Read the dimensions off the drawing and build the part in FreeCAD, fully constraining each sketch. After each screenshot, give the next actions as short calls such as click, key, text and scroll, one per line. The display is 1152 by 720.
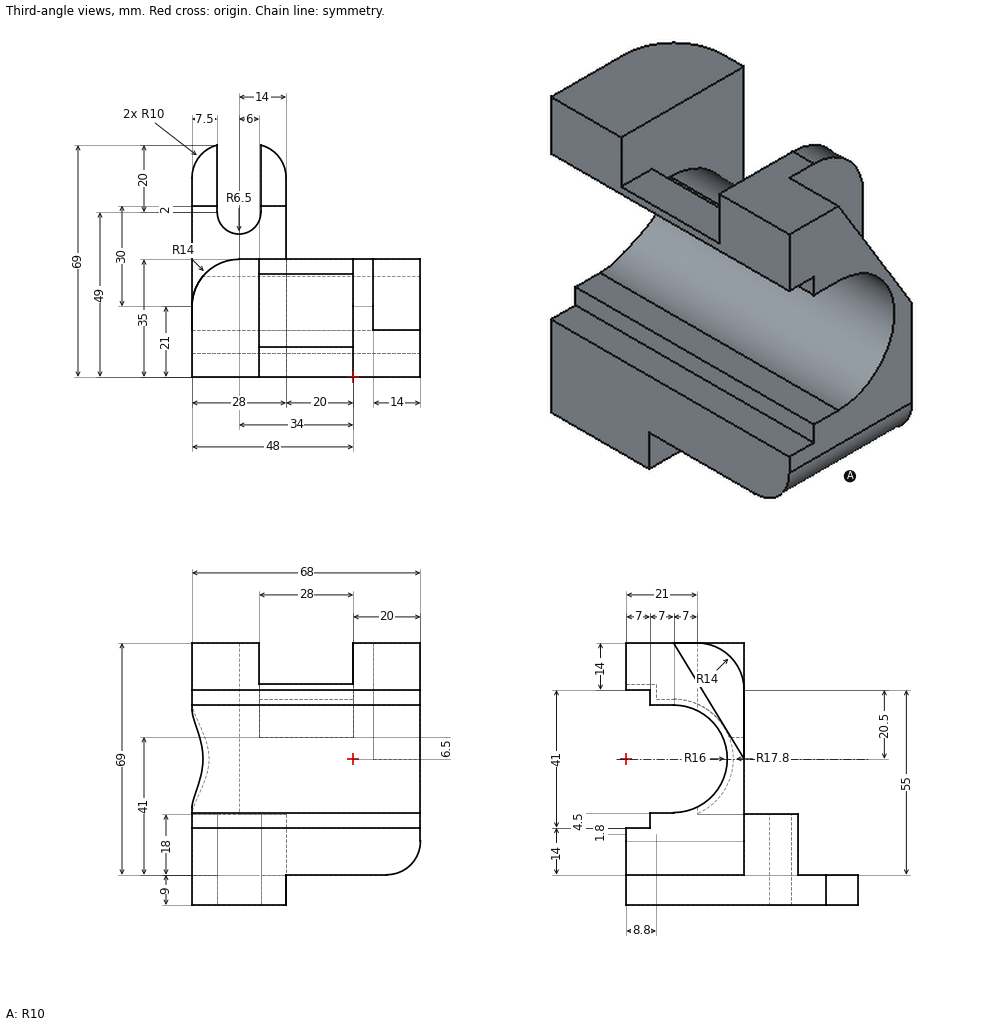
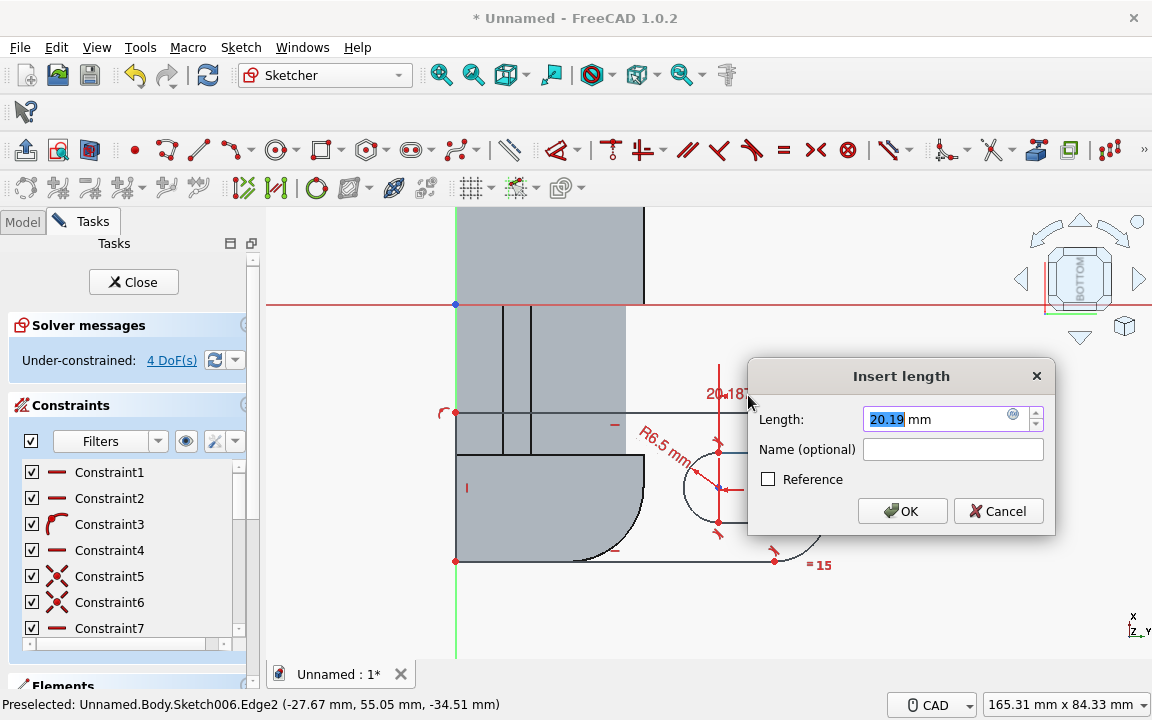
text(20)
key(Return)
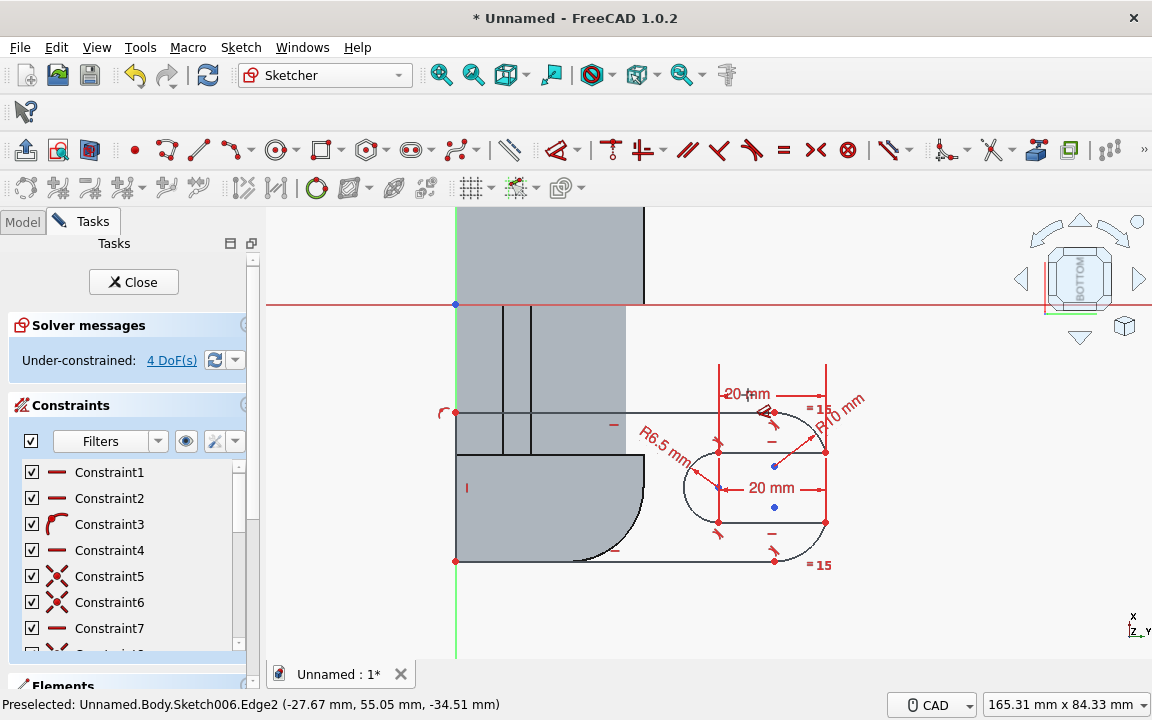
click(456, 458)
click(422, 487)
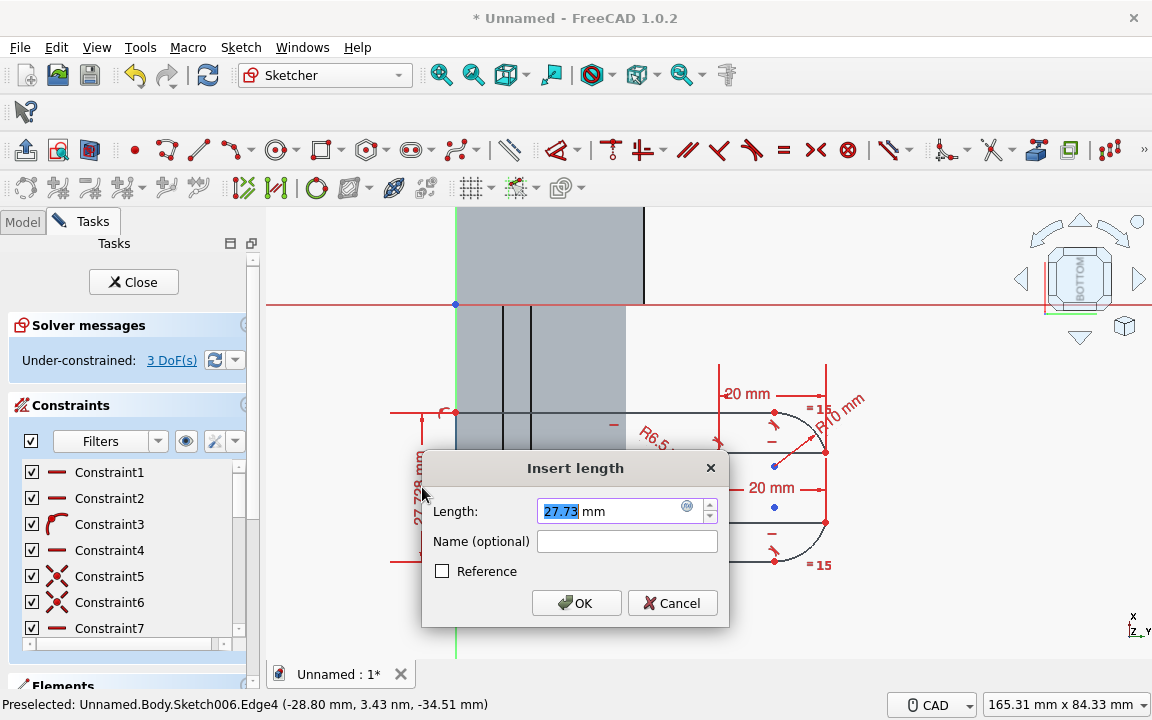
text(28)
key(Return)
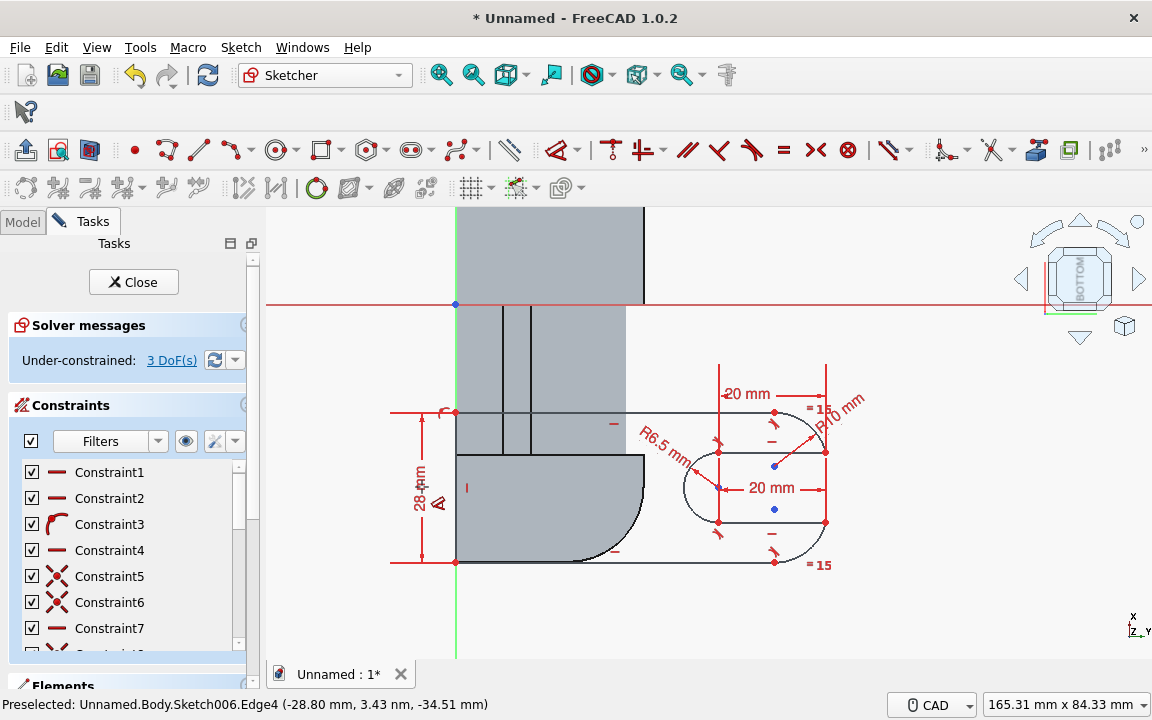
click(826, 523)
click(641, 271)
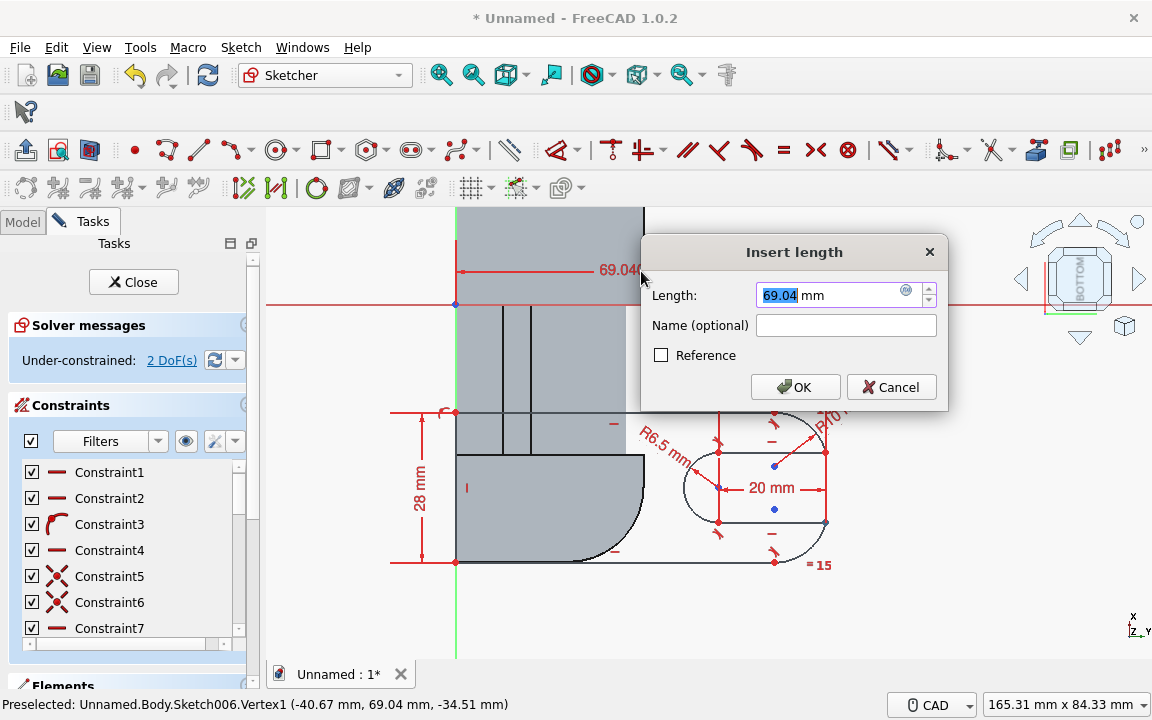
text(69)
key(Return)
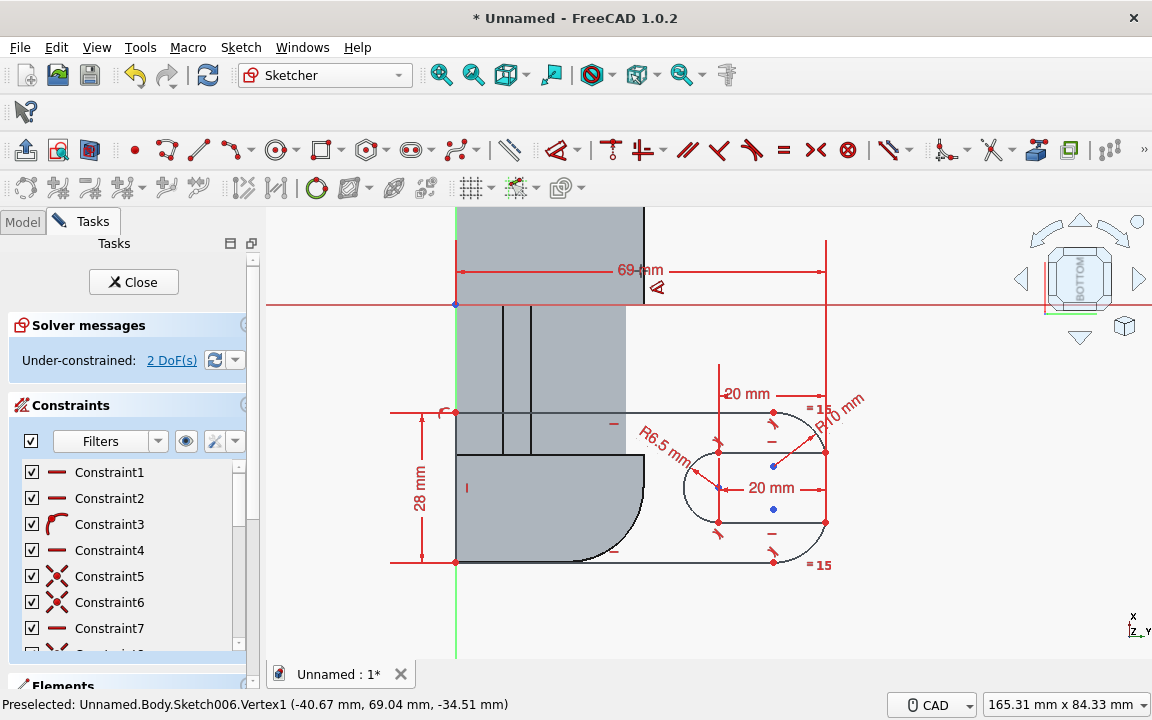
click(774, 413)
click(422, 359)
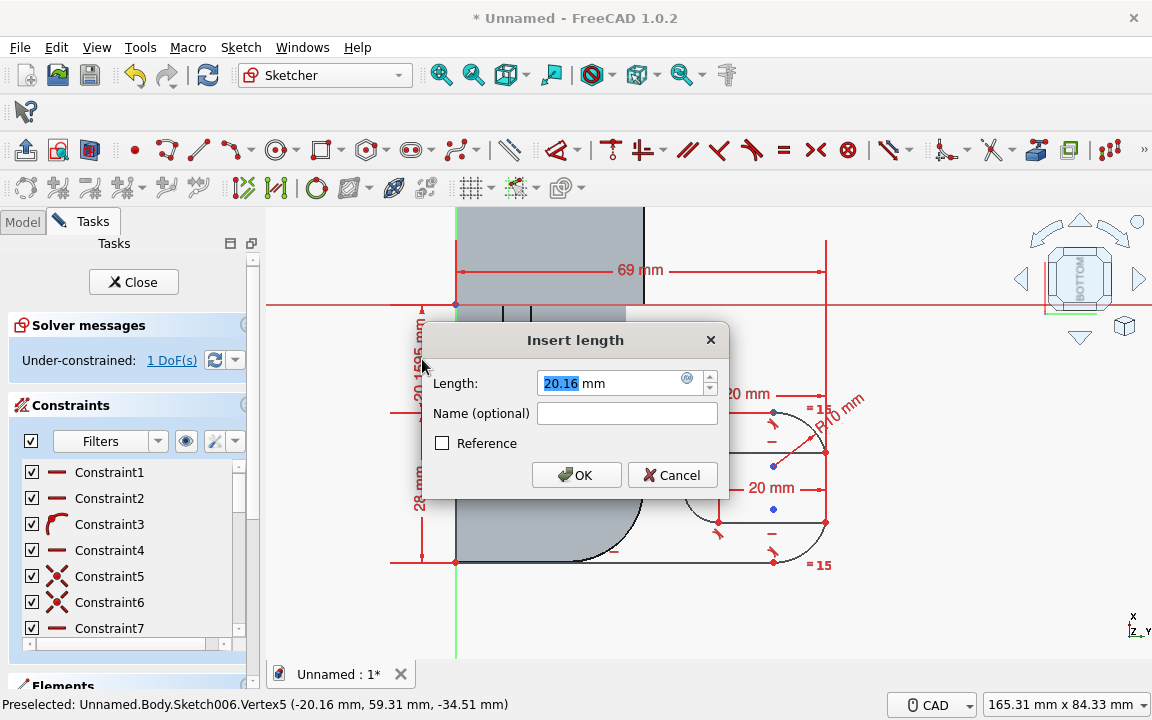
text(20)
key(Return)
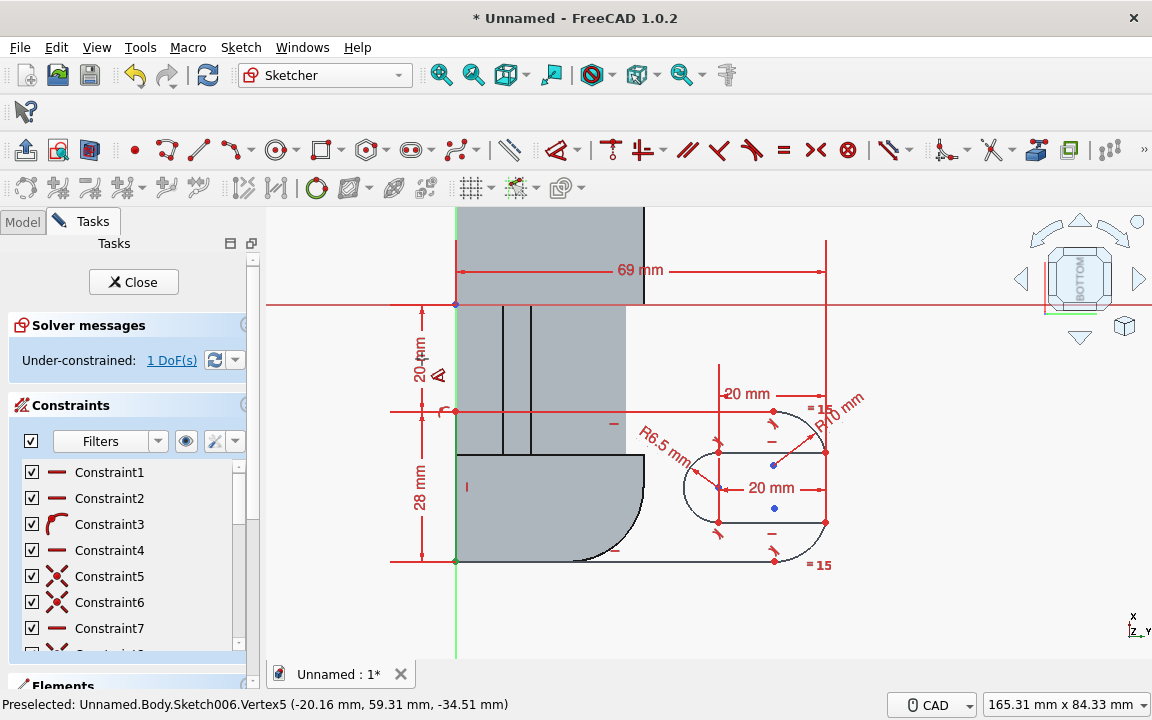
click(719, 488)
click(422, 396)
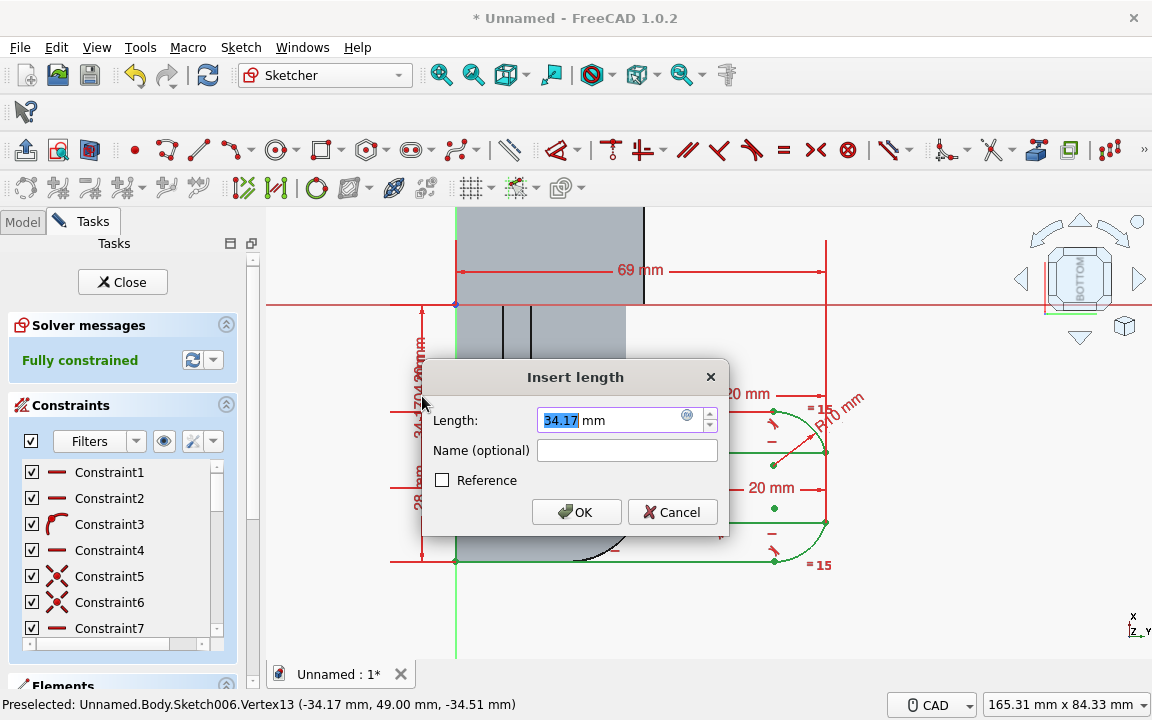
text(34)
key(Return)
key(Escape)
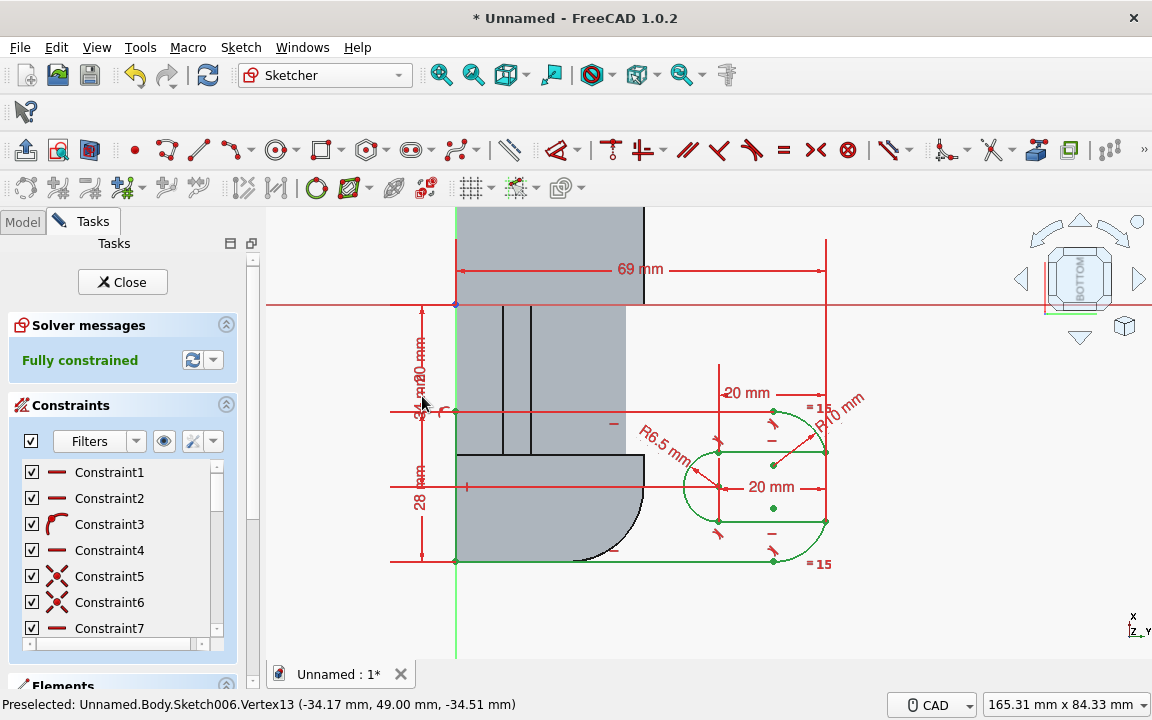
click(123, 282)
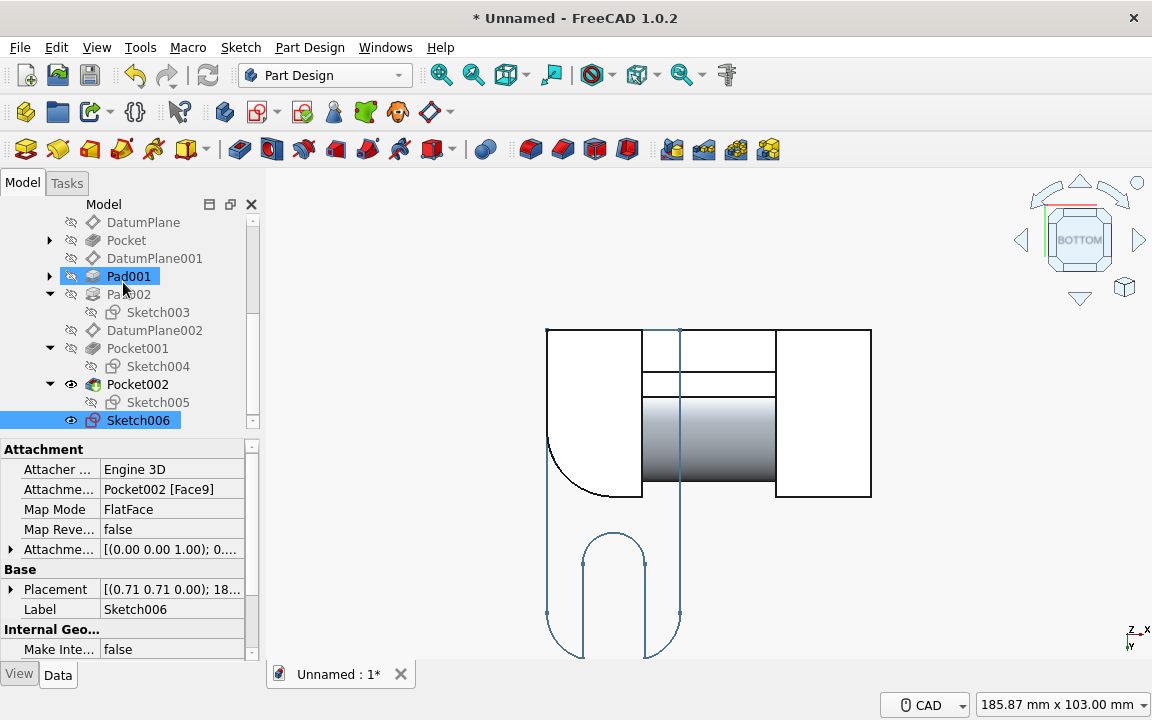
click(26, 150)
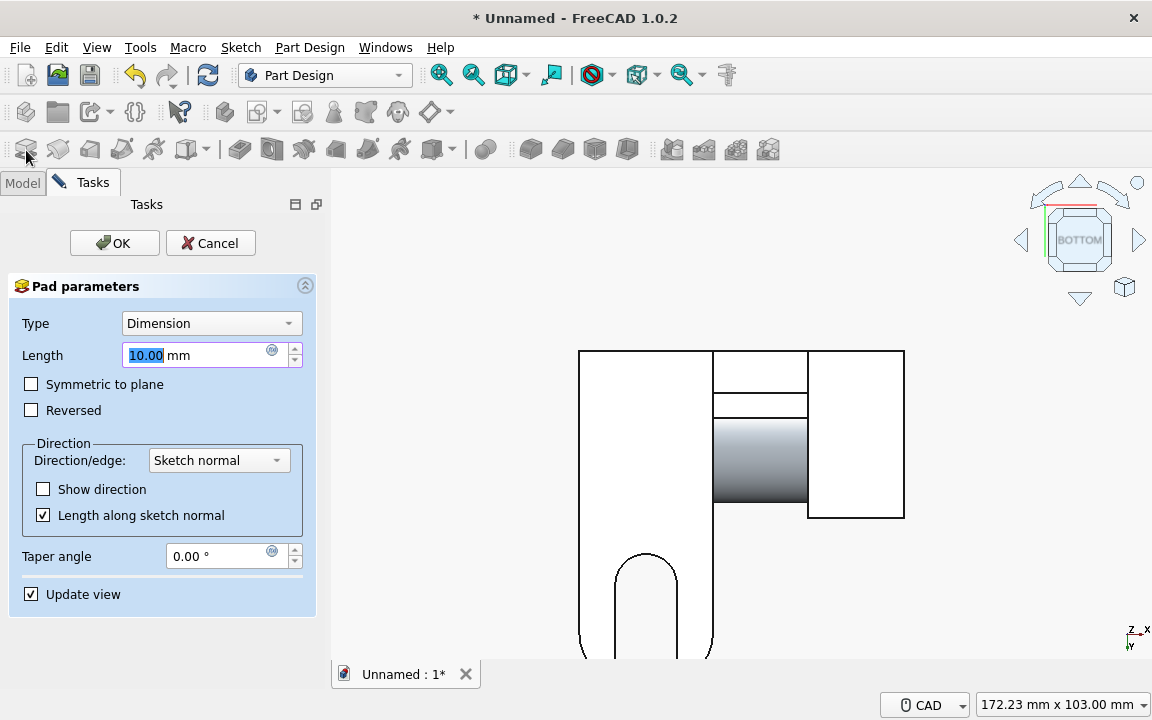
text(9)
key(Tab)